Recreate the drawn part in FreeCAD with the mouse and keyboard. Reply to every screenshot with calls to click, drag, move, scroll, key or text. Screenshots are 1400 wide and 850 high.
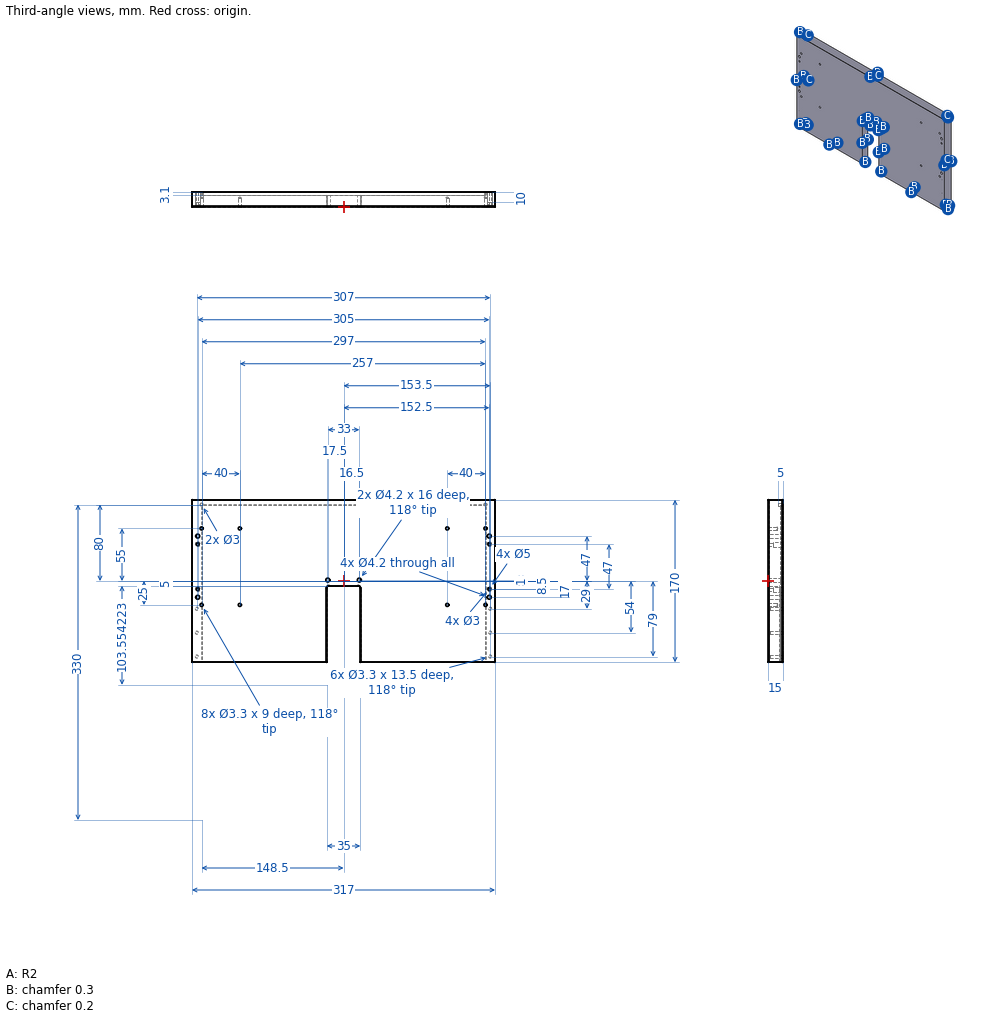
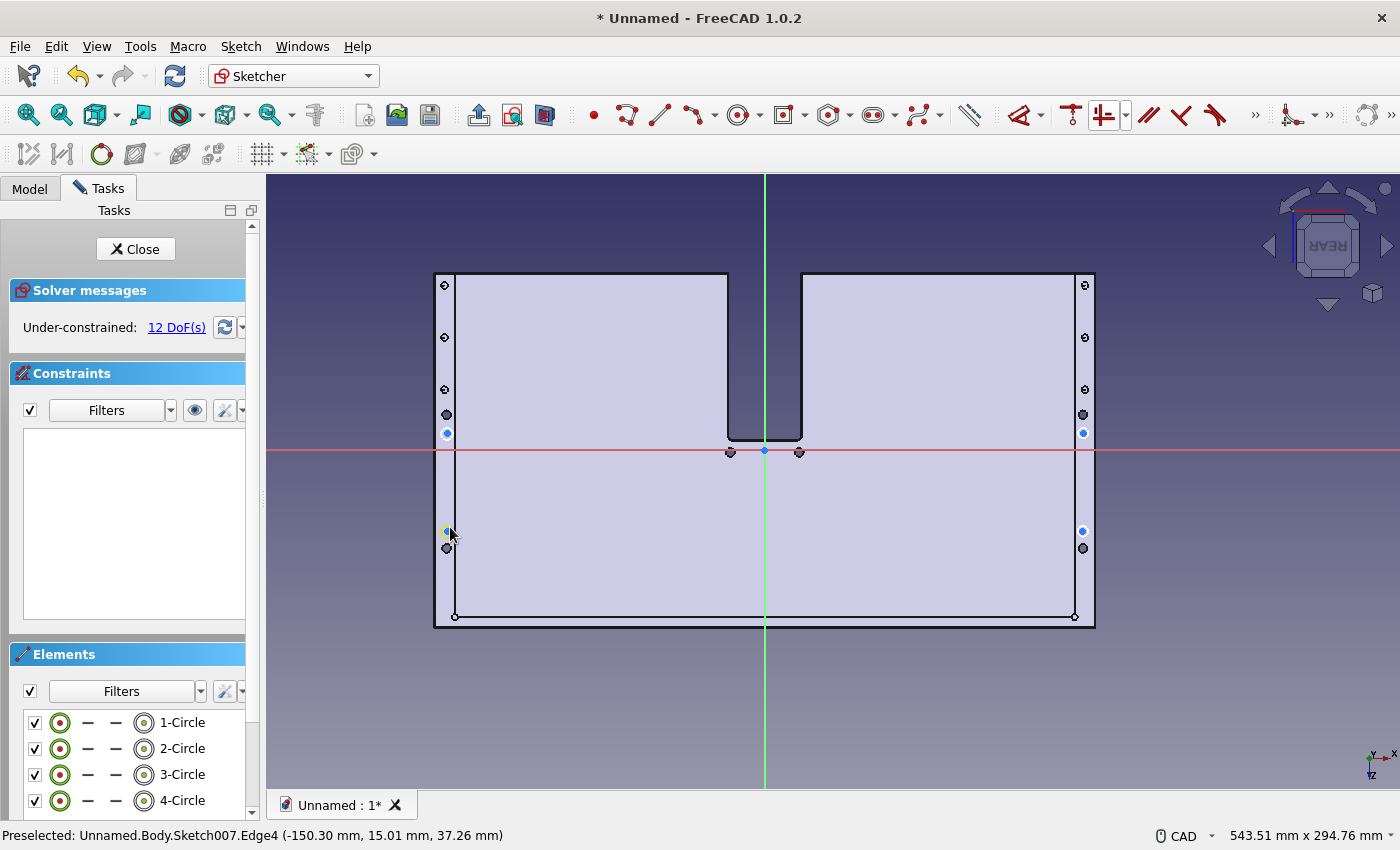
scroll(1087, 429, up, 5)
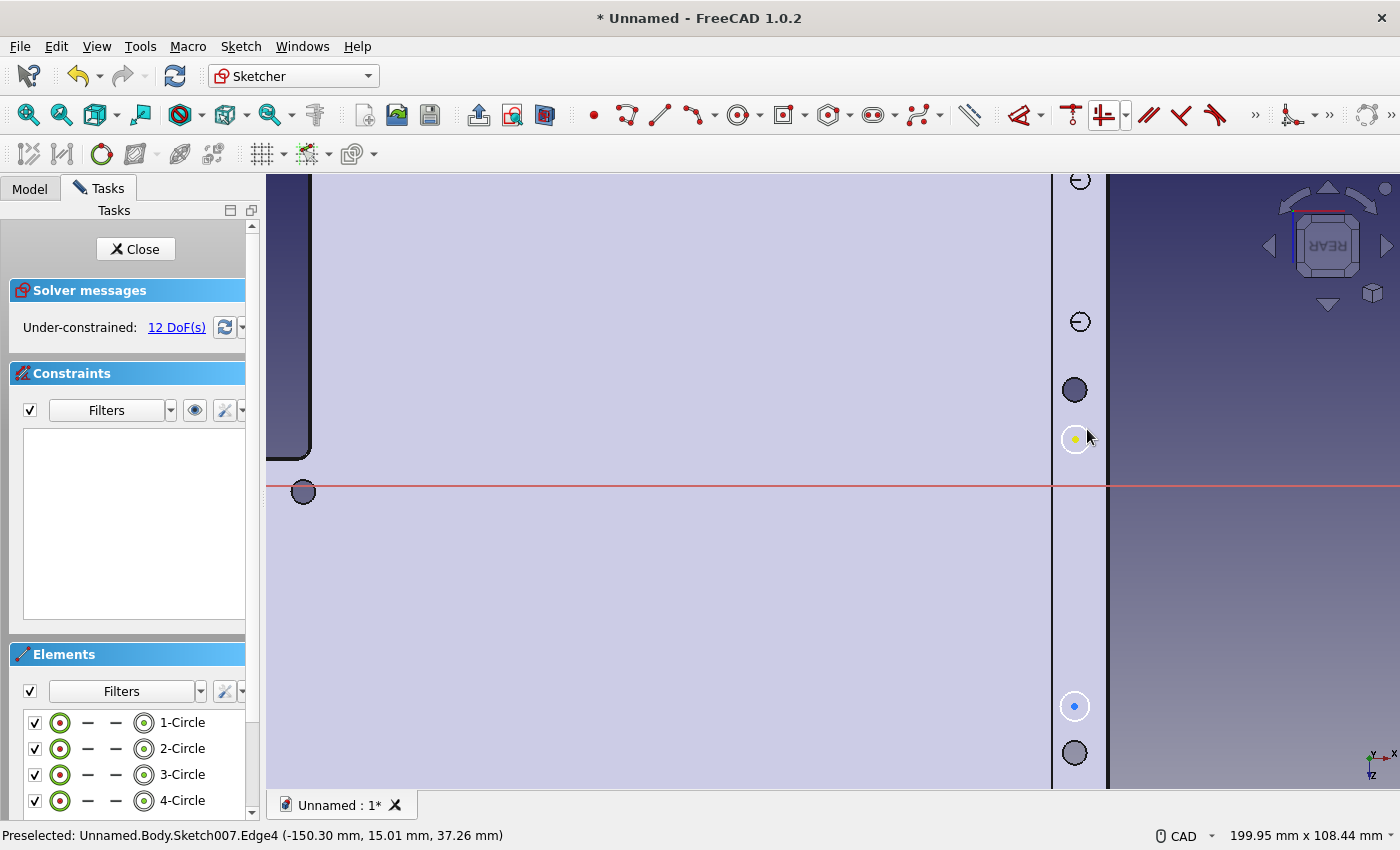
click(1086, 430)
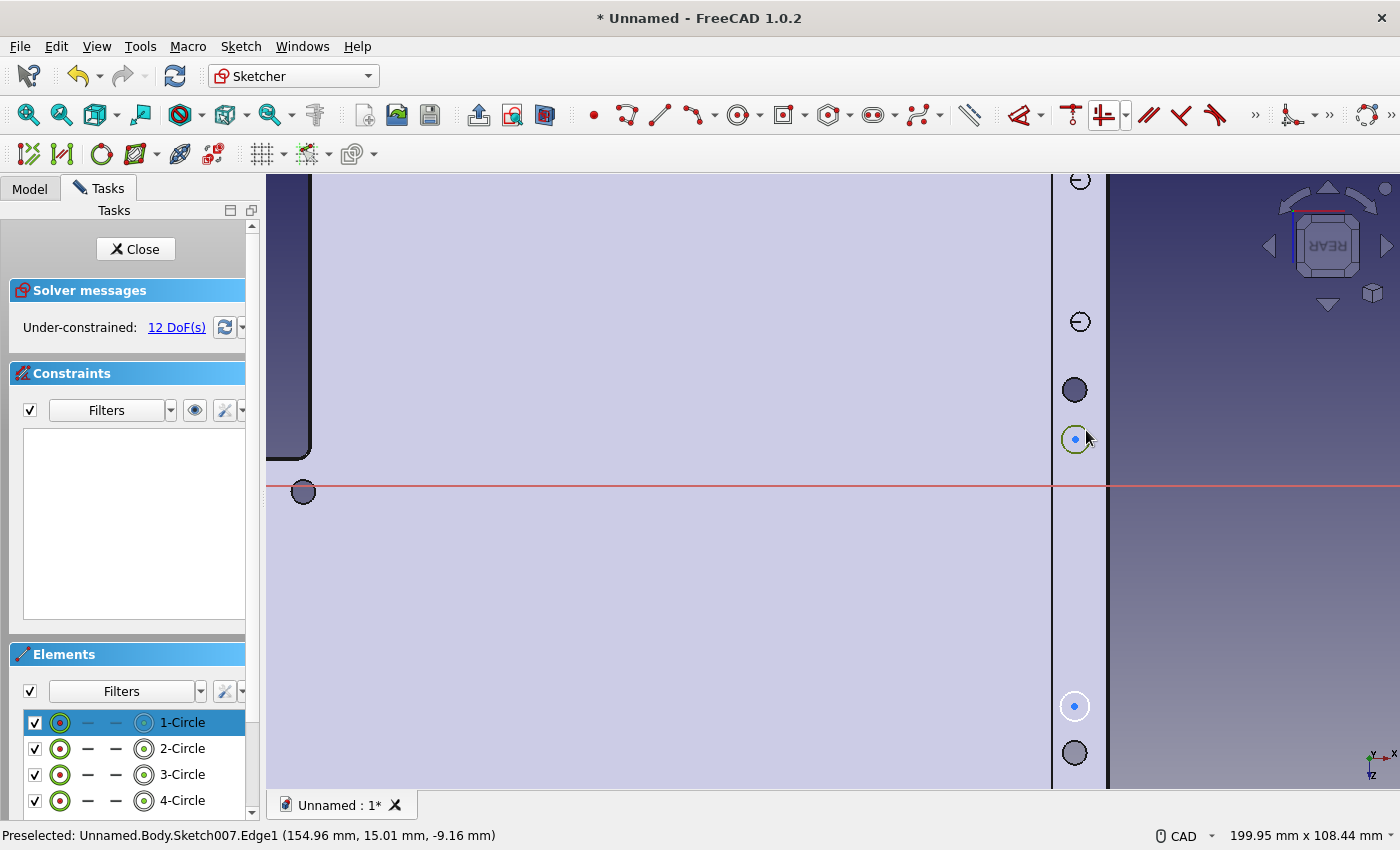
click(1085, 696)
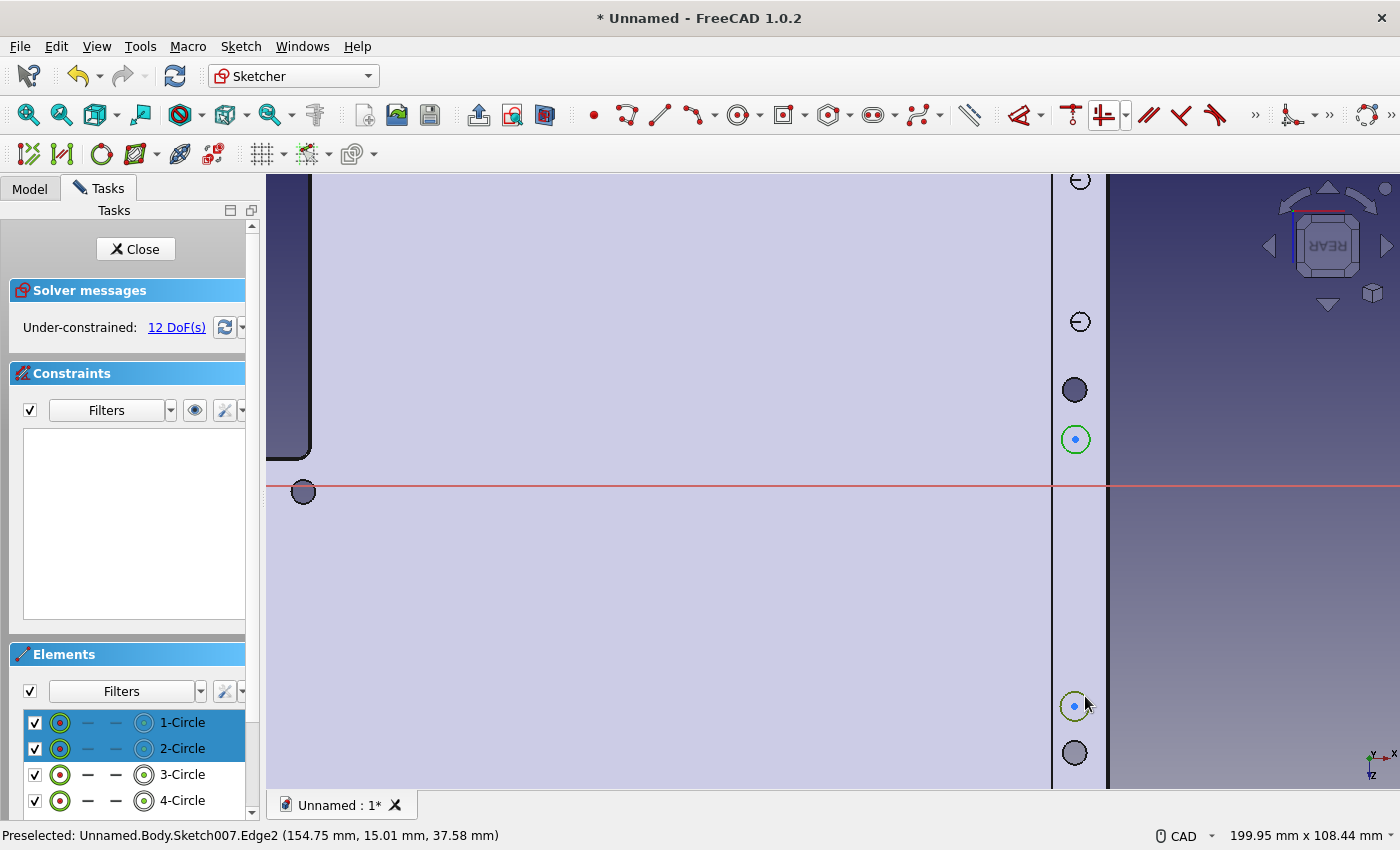
scroll(1087, 429, down, 5)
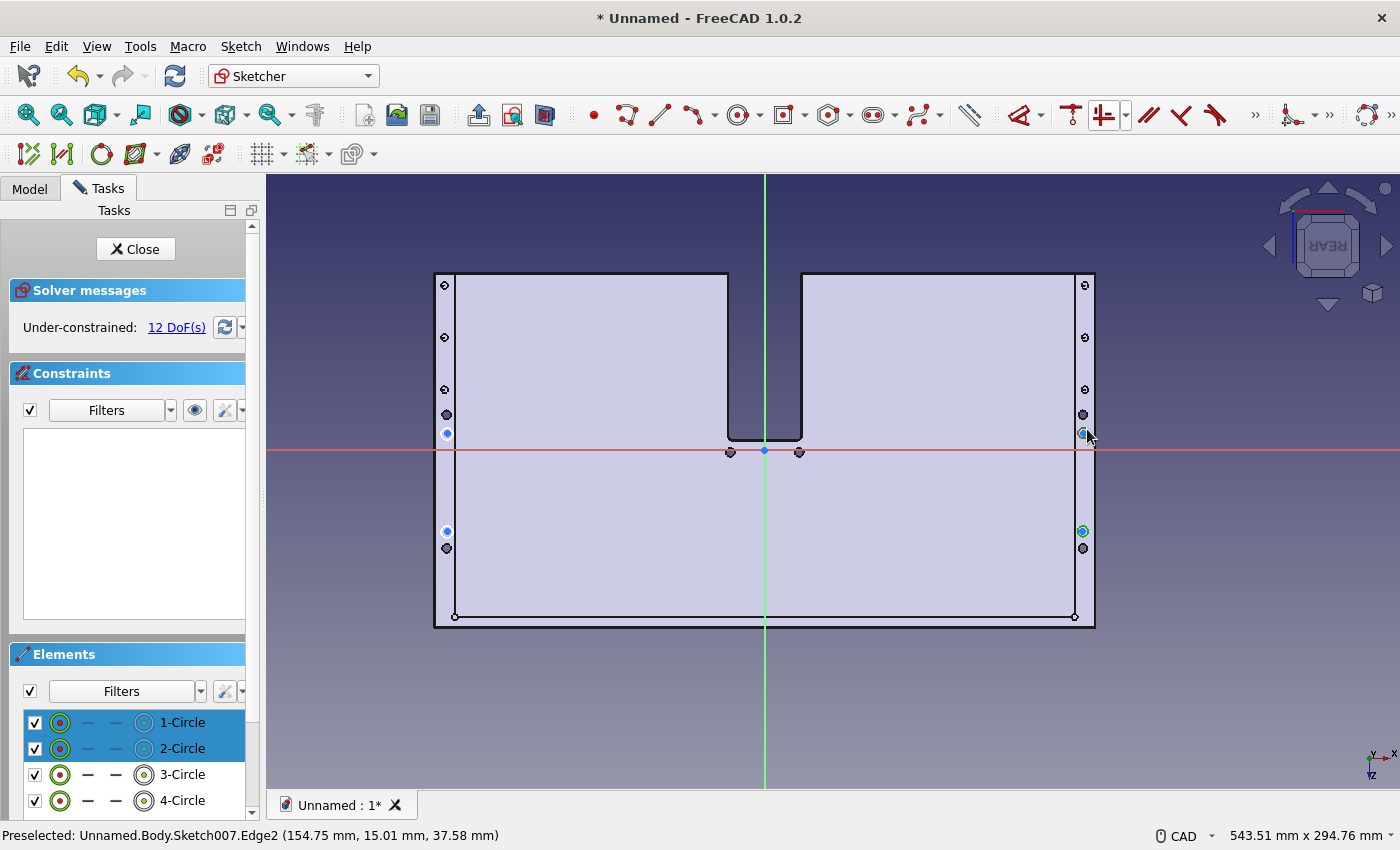
scroll(451, 430, up, 5)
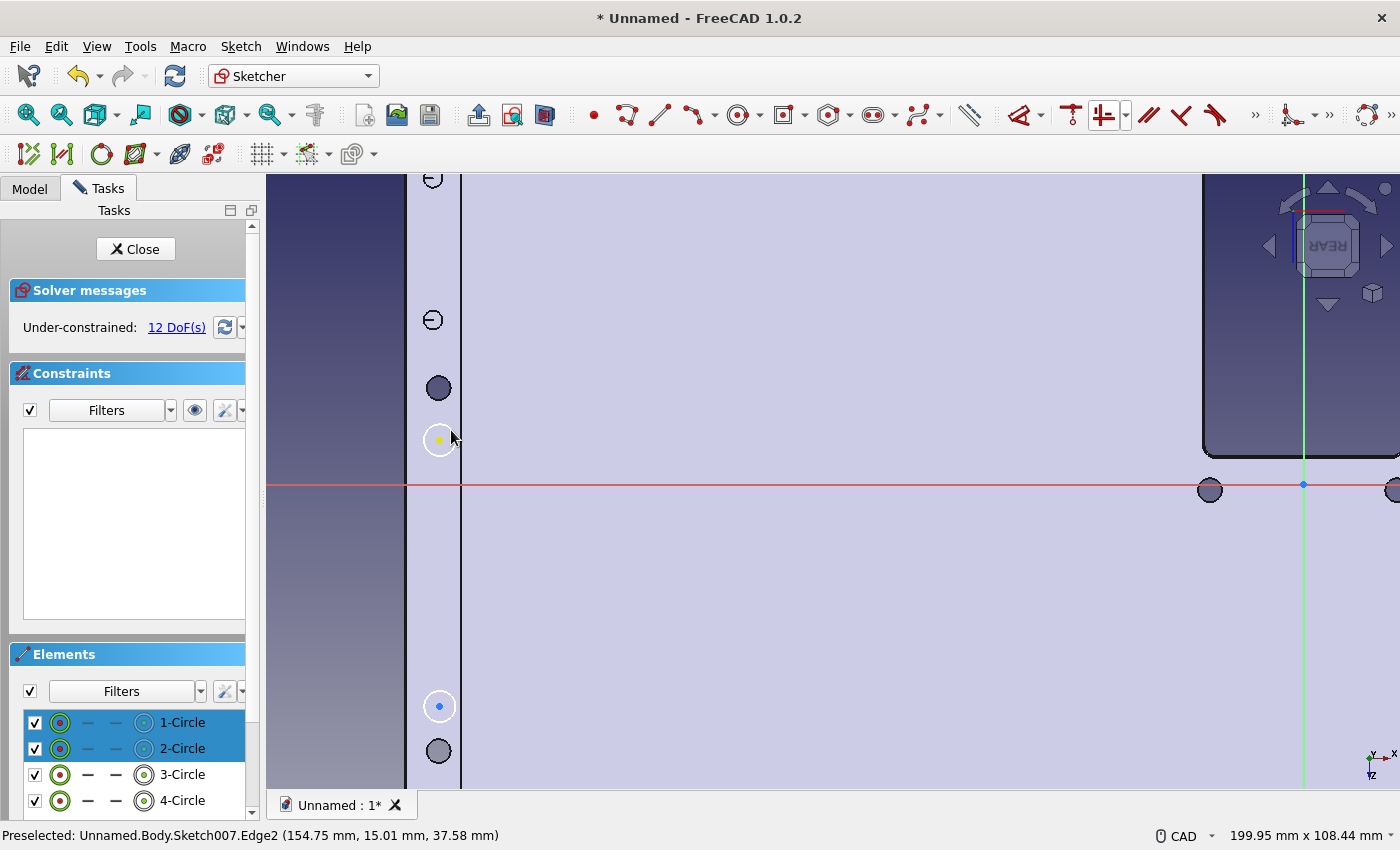
click(451, 429)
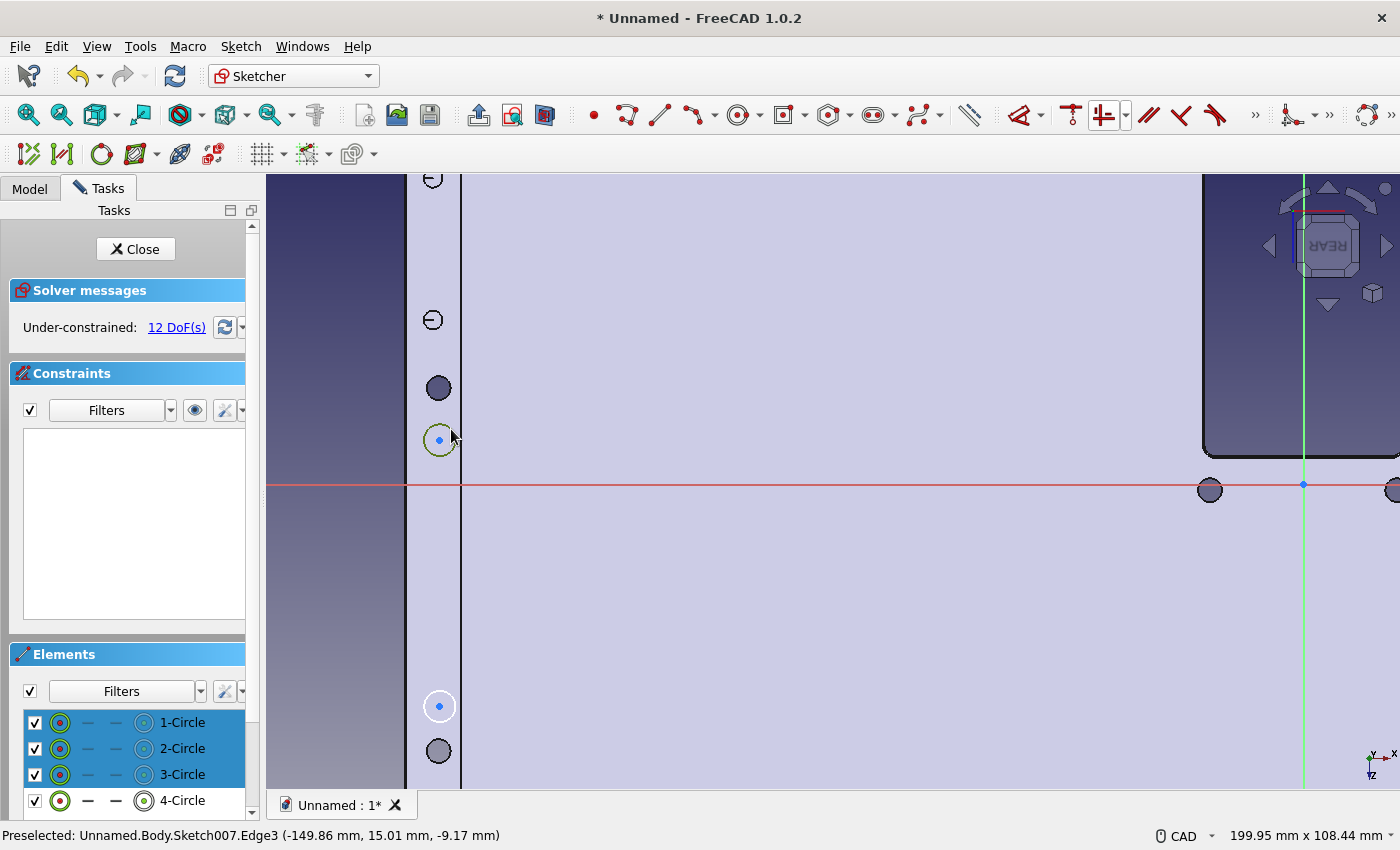
click(451, 696)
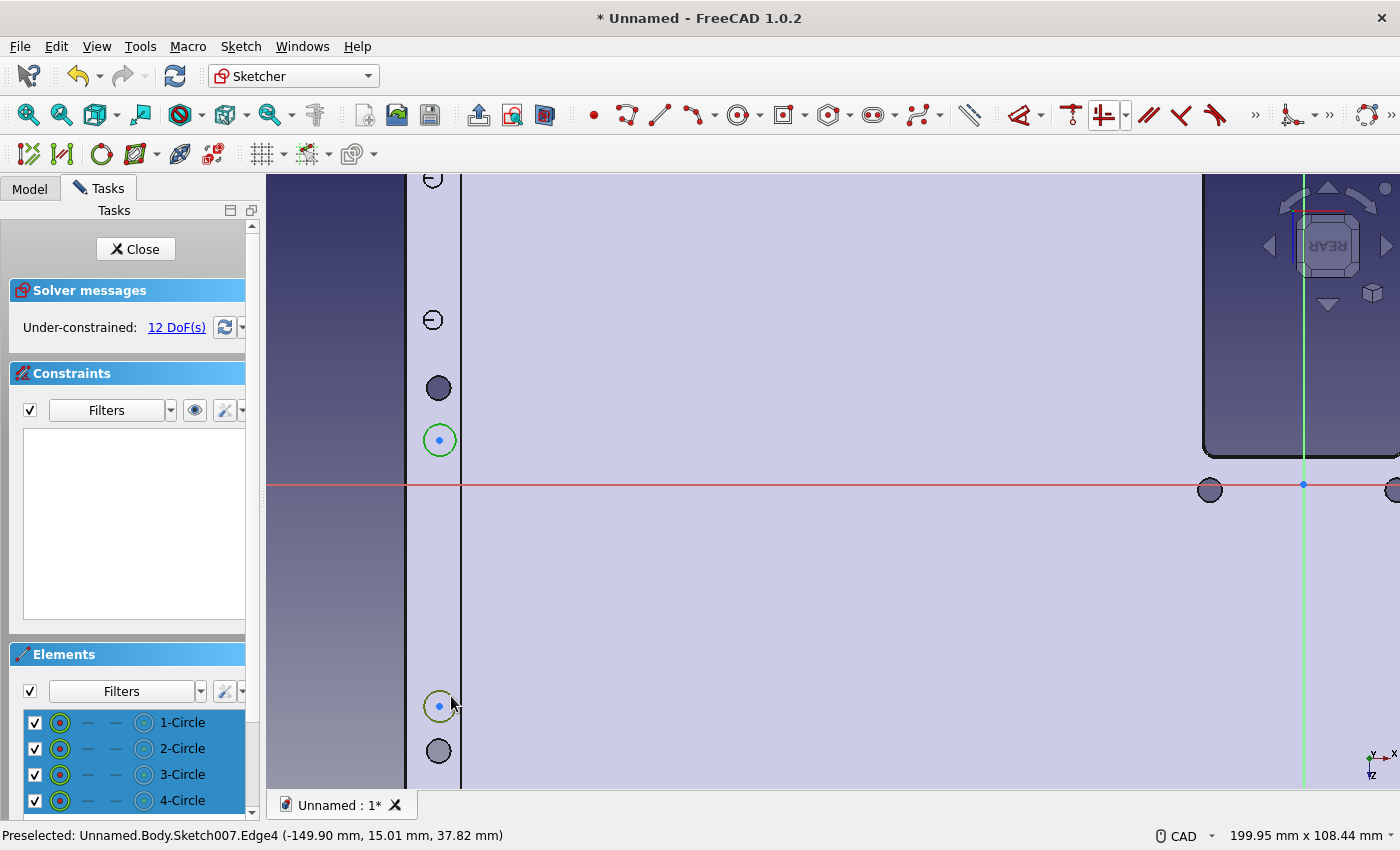
key(e)